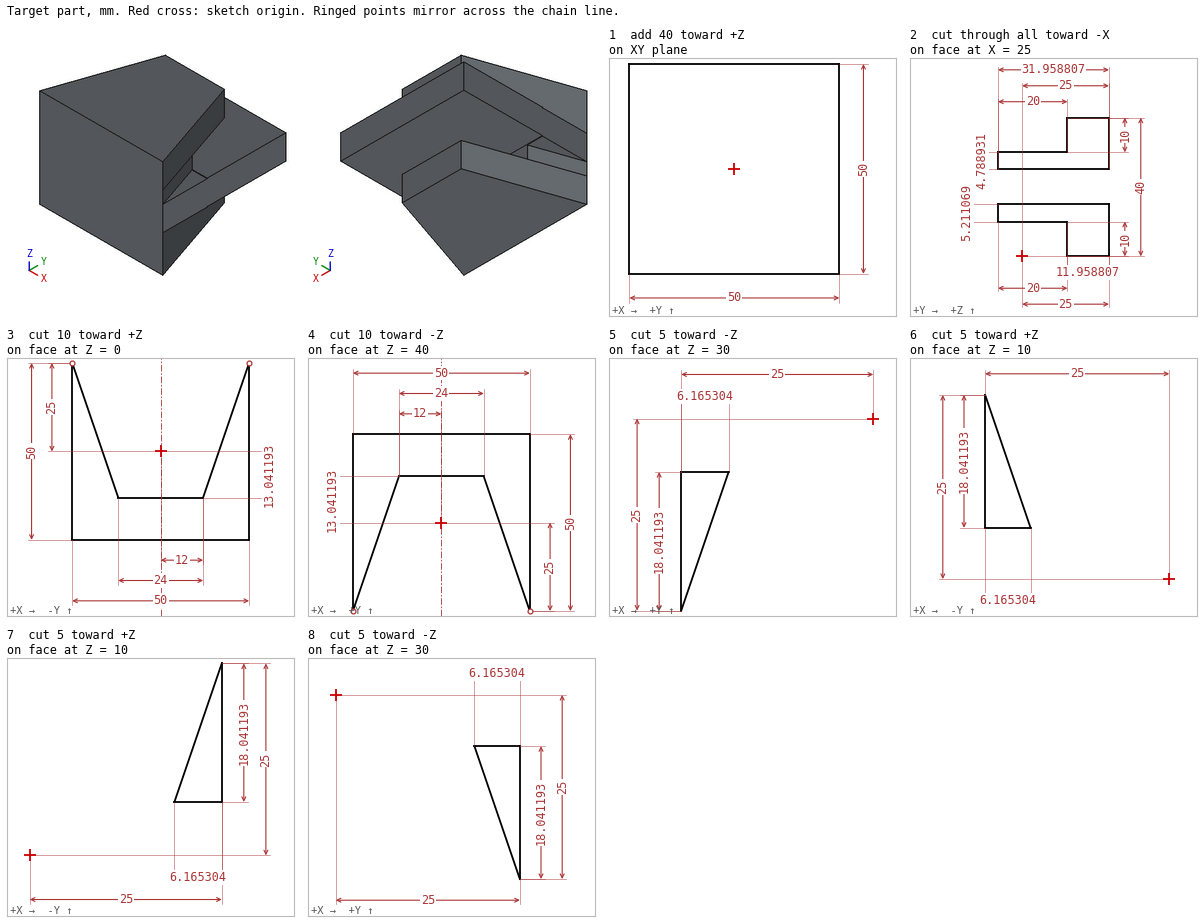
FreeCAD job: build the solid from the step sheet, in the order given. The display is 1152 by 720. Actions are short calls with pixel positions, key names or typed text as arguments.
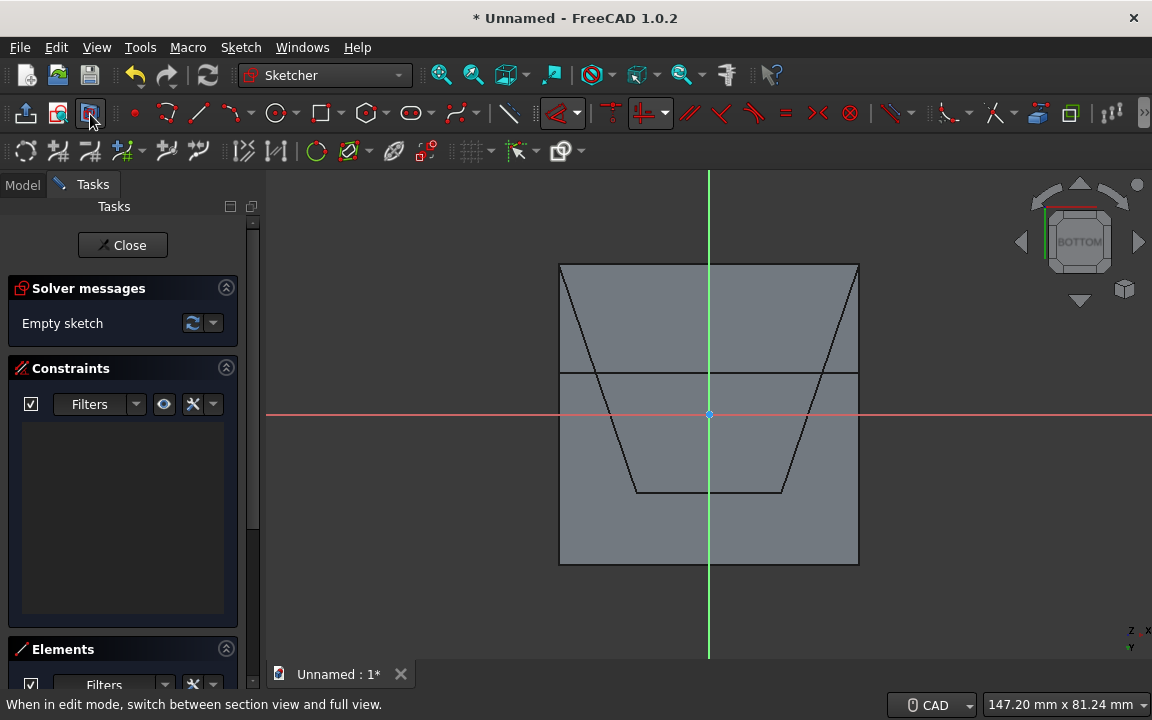
scroll(628, 278, up, 4)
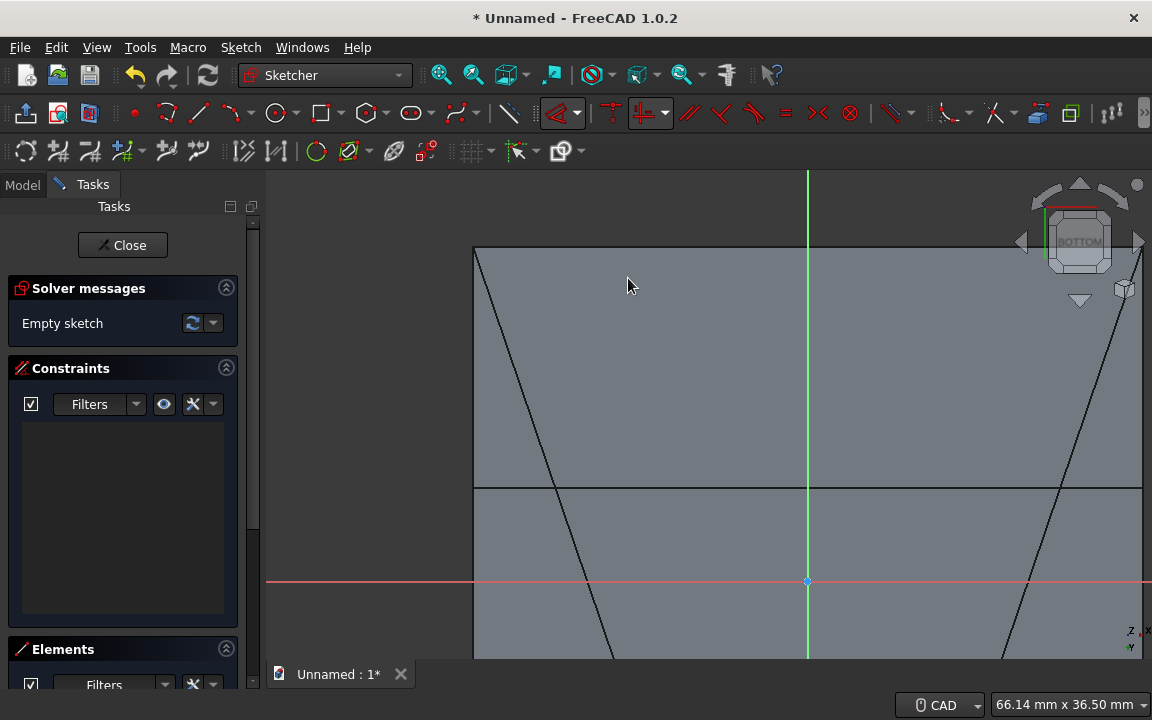
key(g)
key(m)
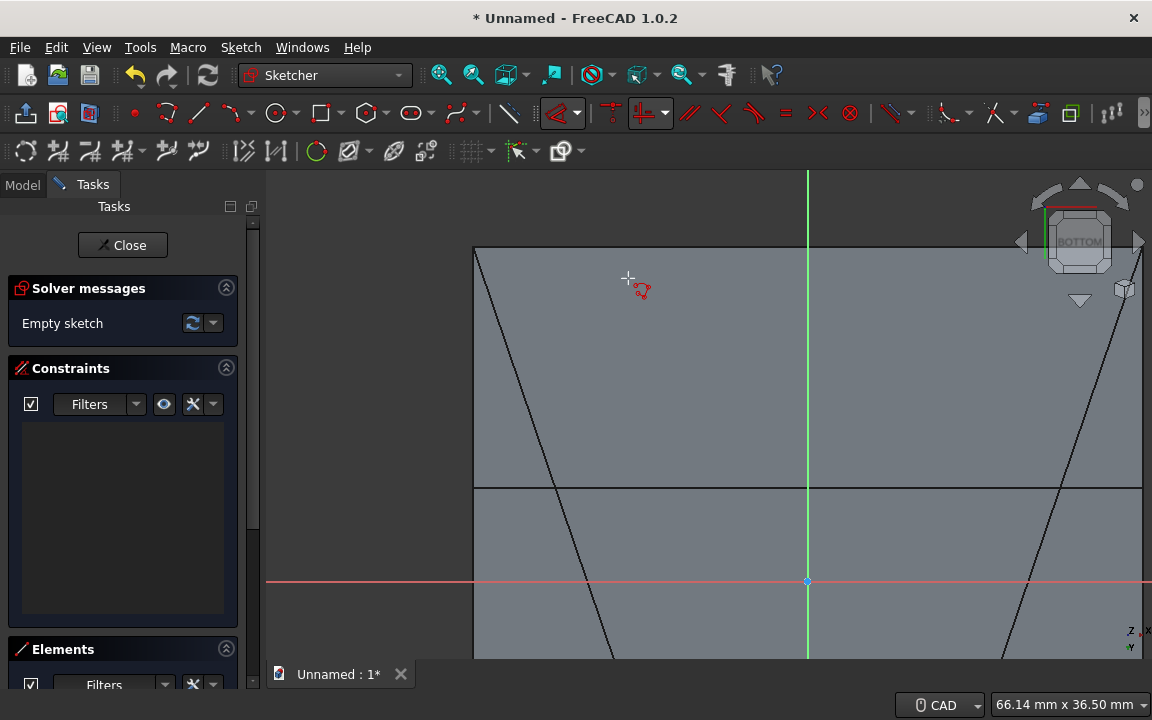
click(555, 488)
click(473, 247)
click(473, 488)
click(555, 489)
key(Escape)
key(Escape)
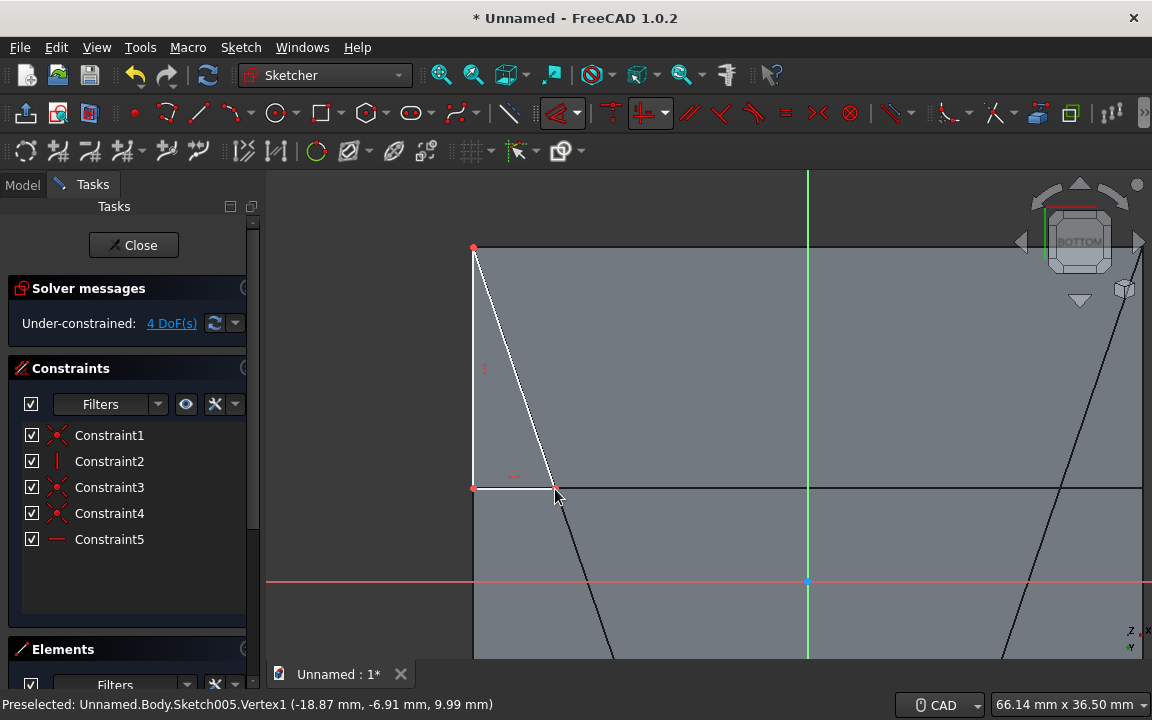
click(473, 248)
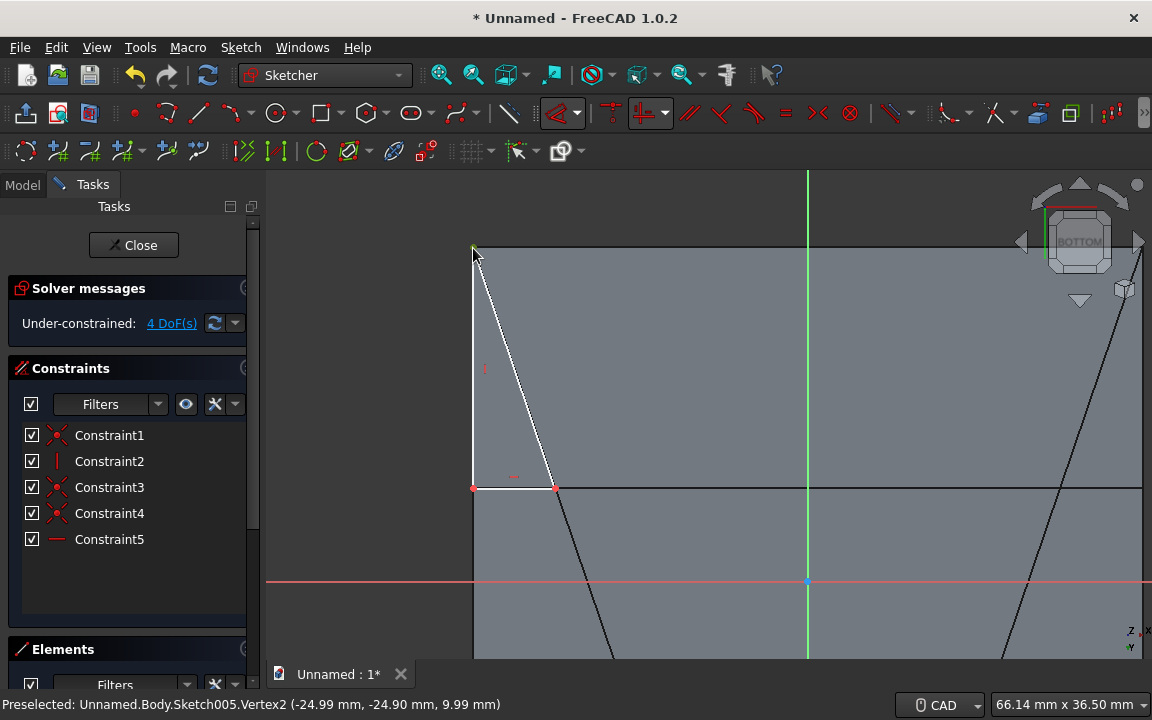
key(l)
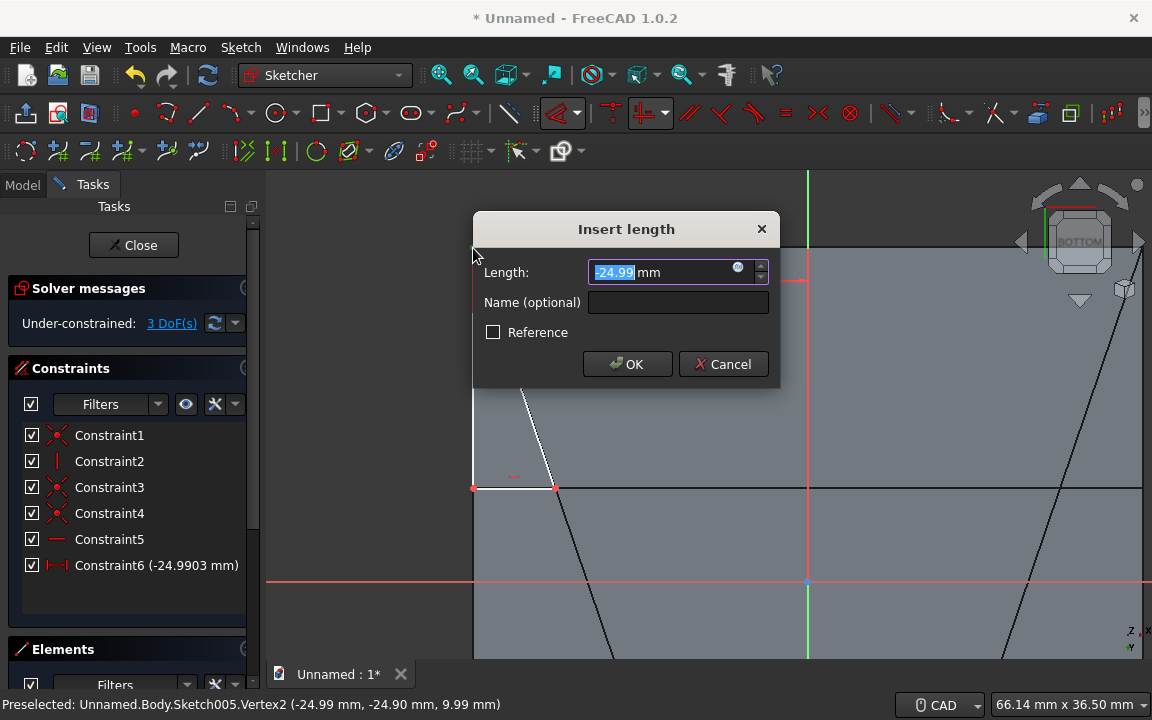
text(-25)
key(Return)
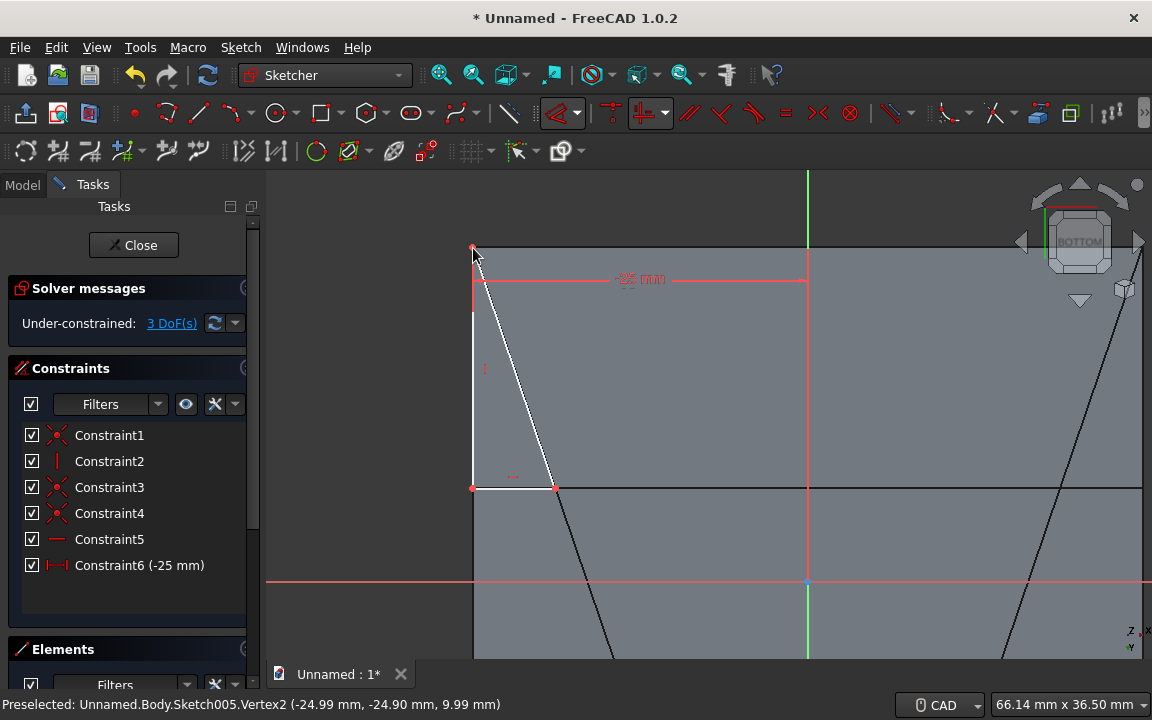
click(473, 248)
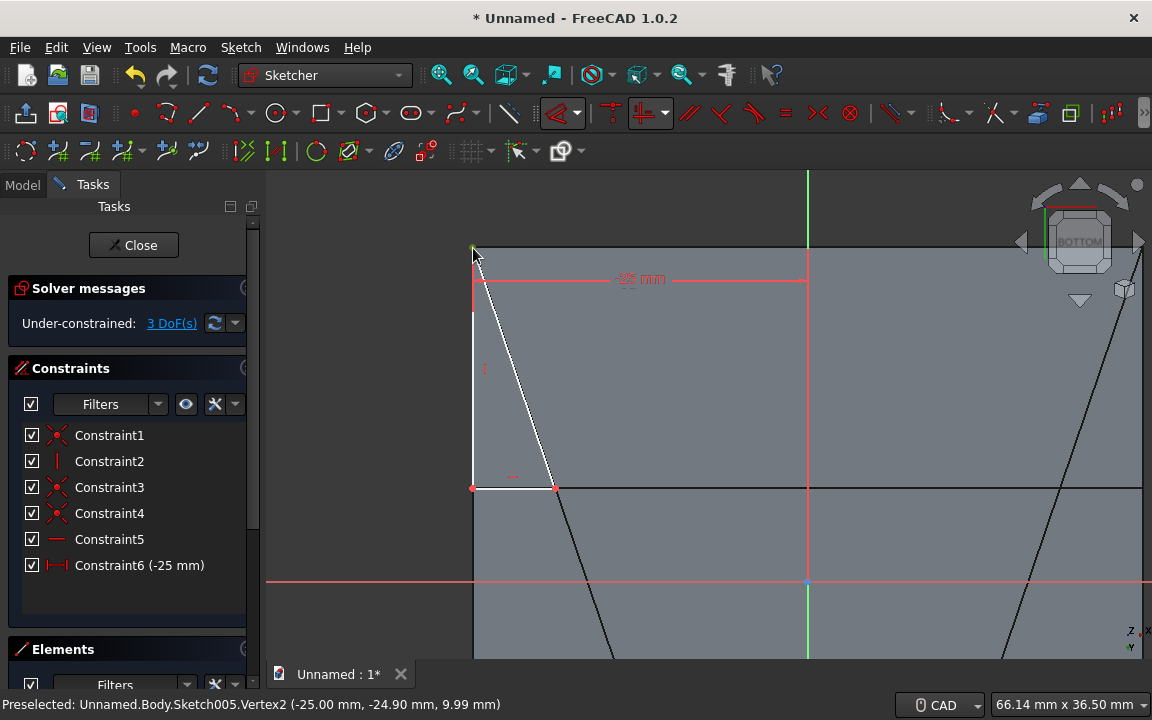
key(i)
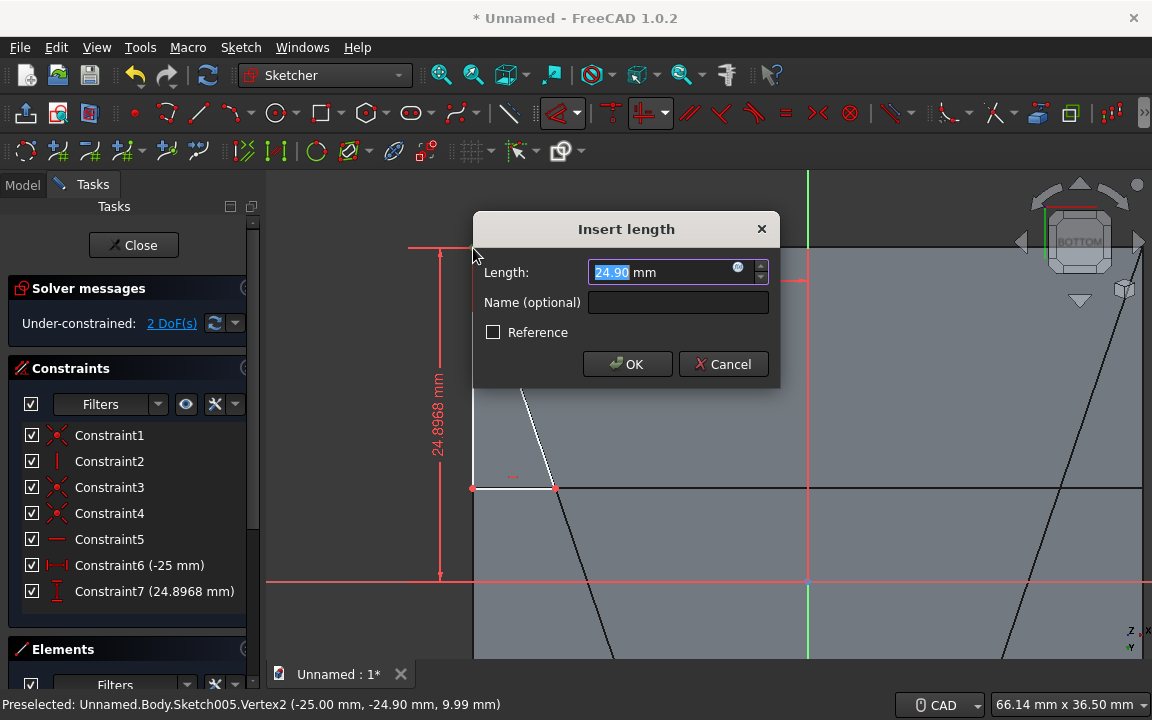
text(25)
key(Return)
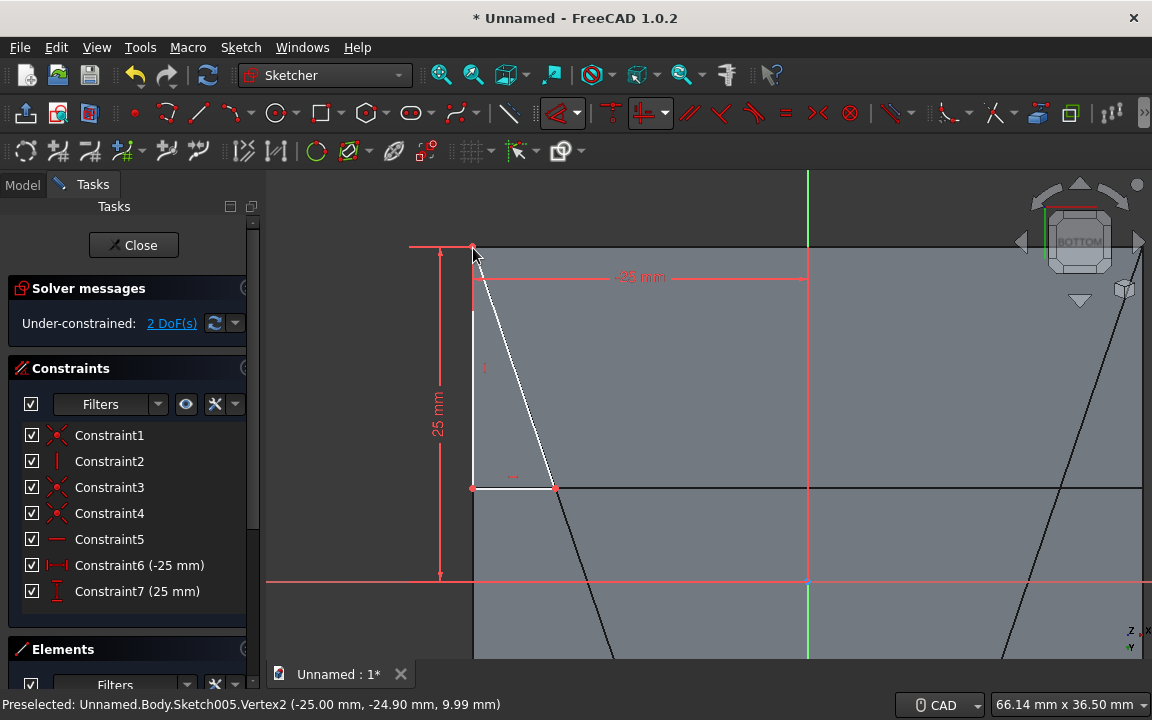
click(498, 489)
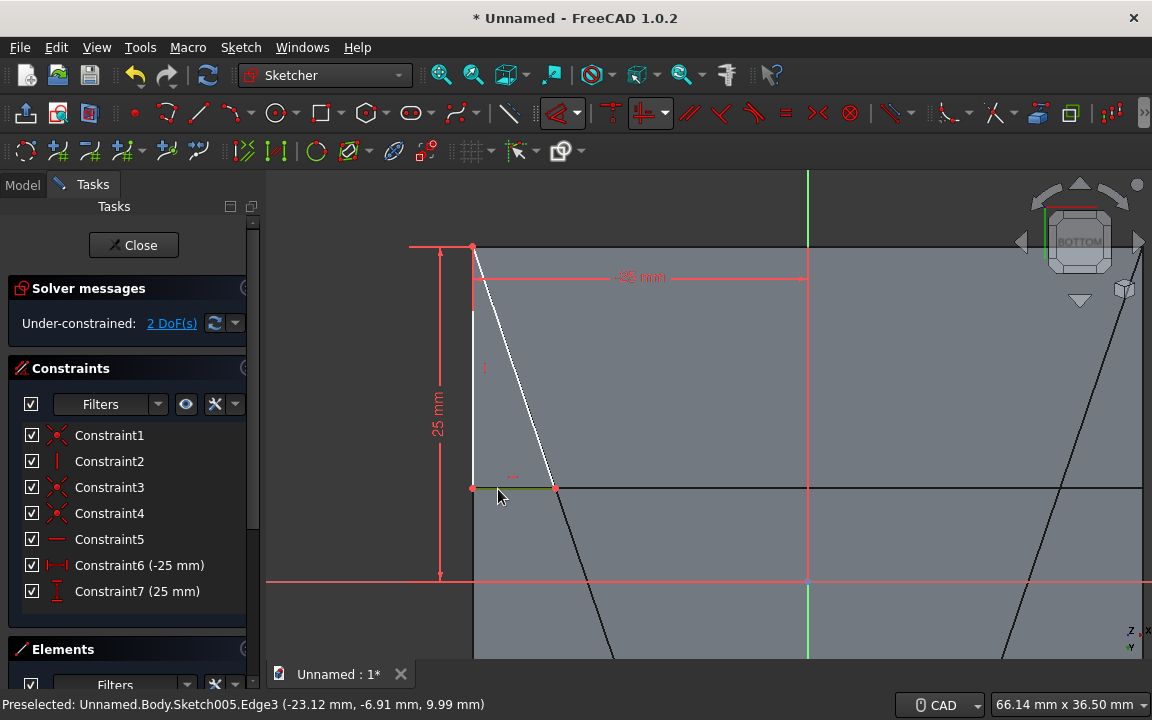
key(l)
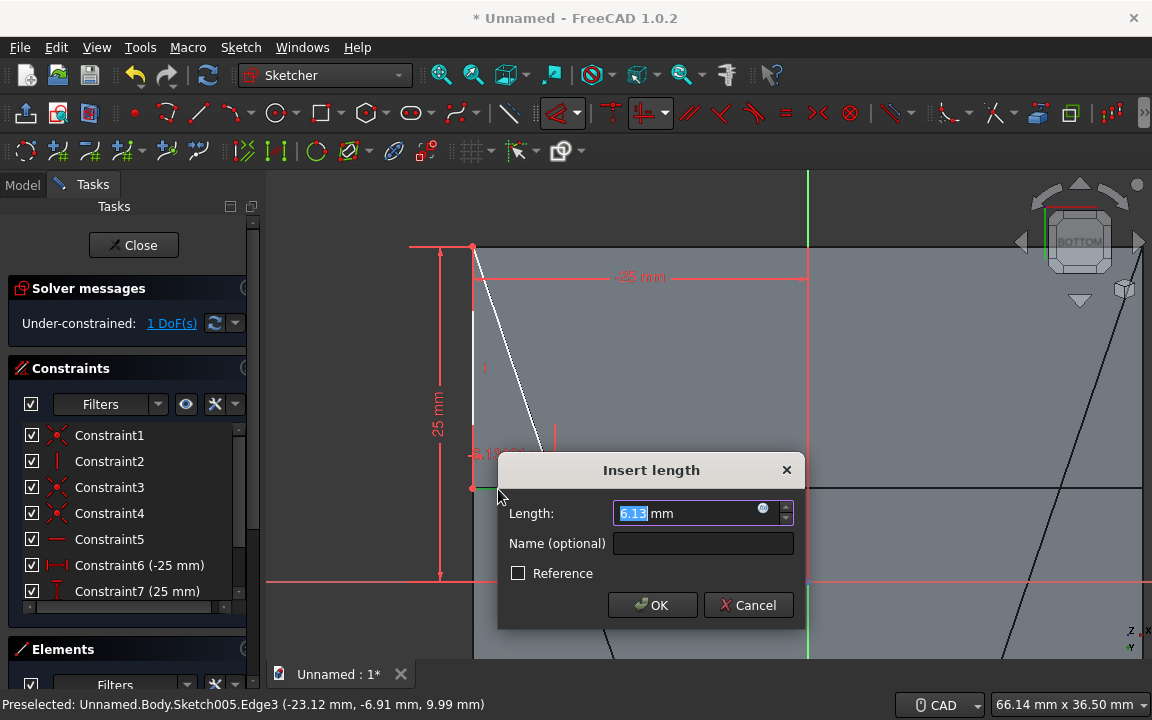
text(6.165304)
key(Return)